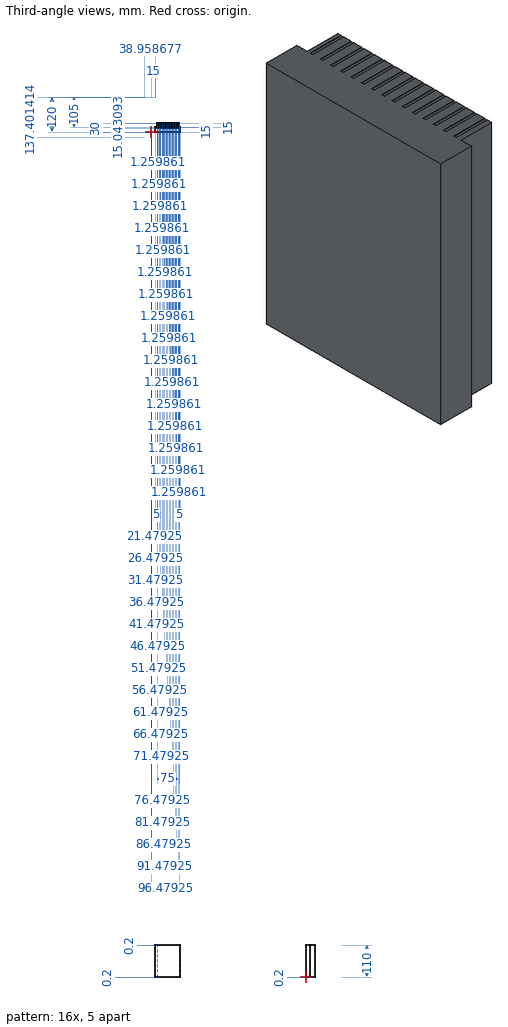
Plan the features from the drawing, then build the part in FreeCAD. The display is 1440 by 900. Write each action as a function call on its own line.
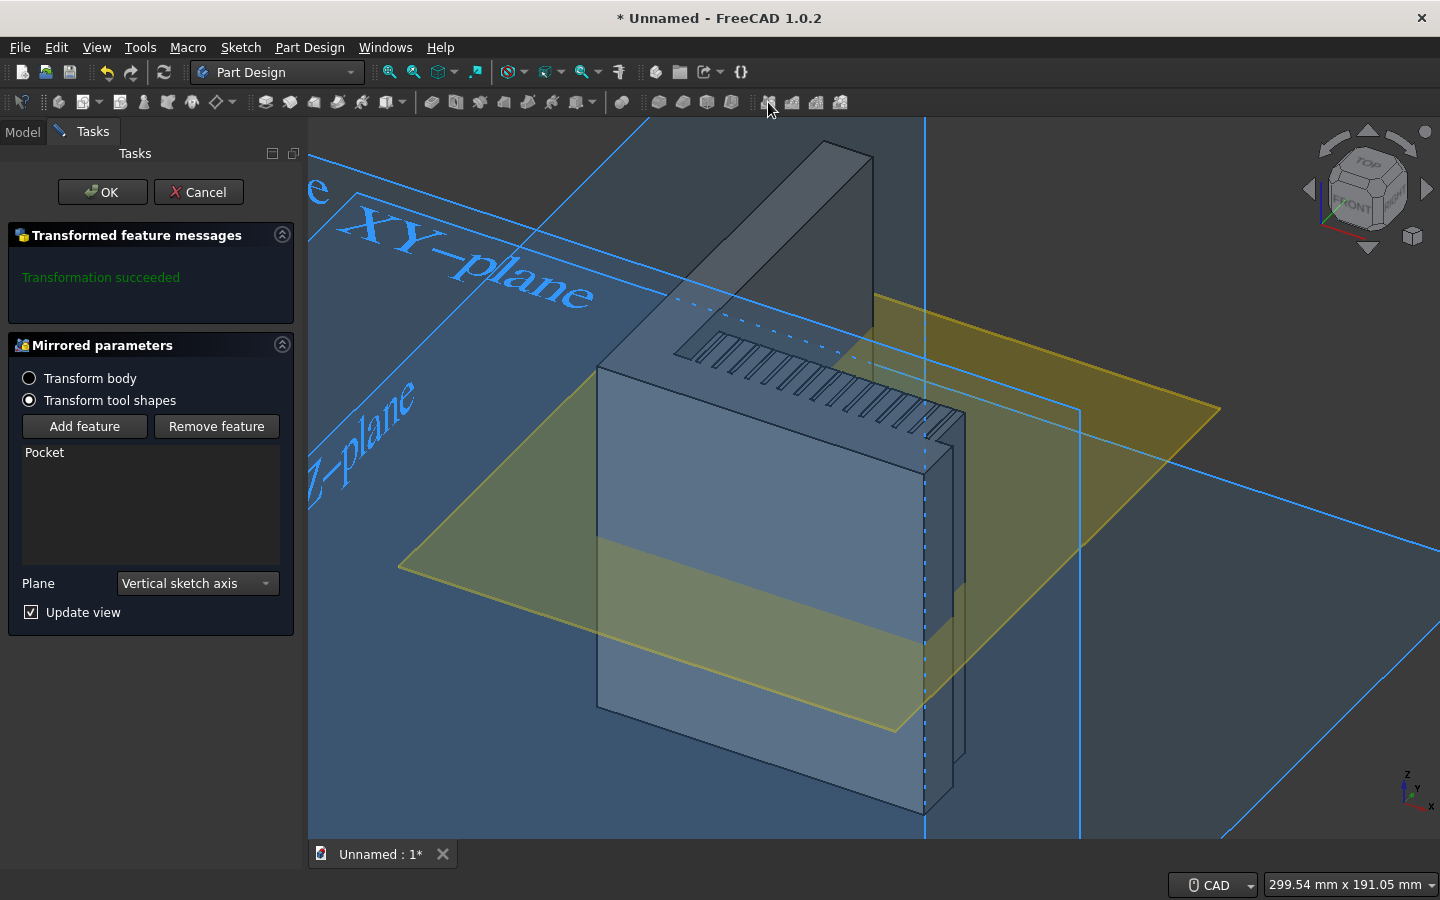
click(198, 584)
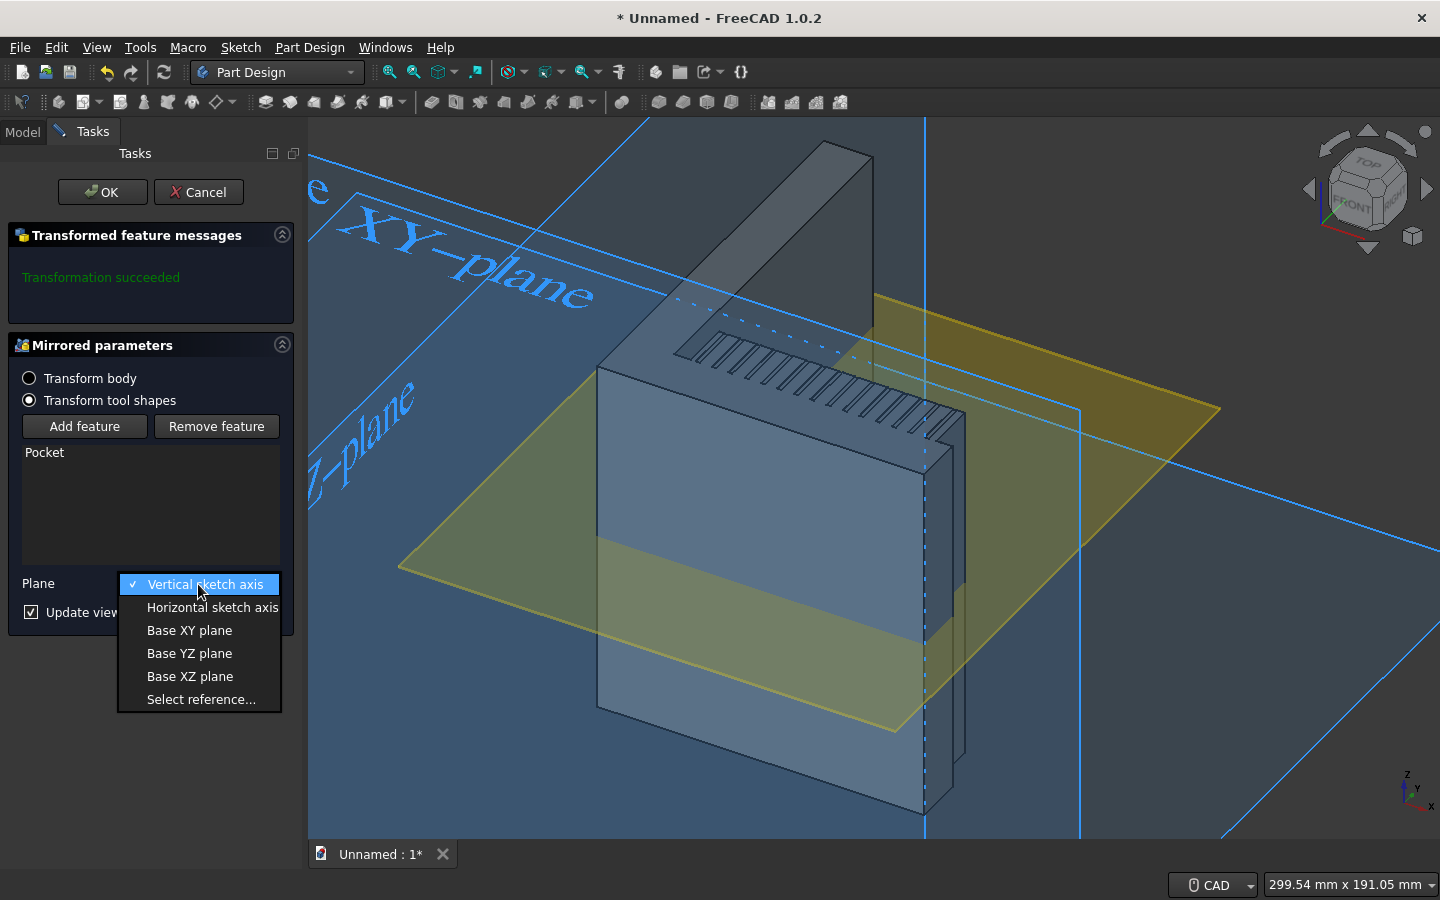
click(198, 700)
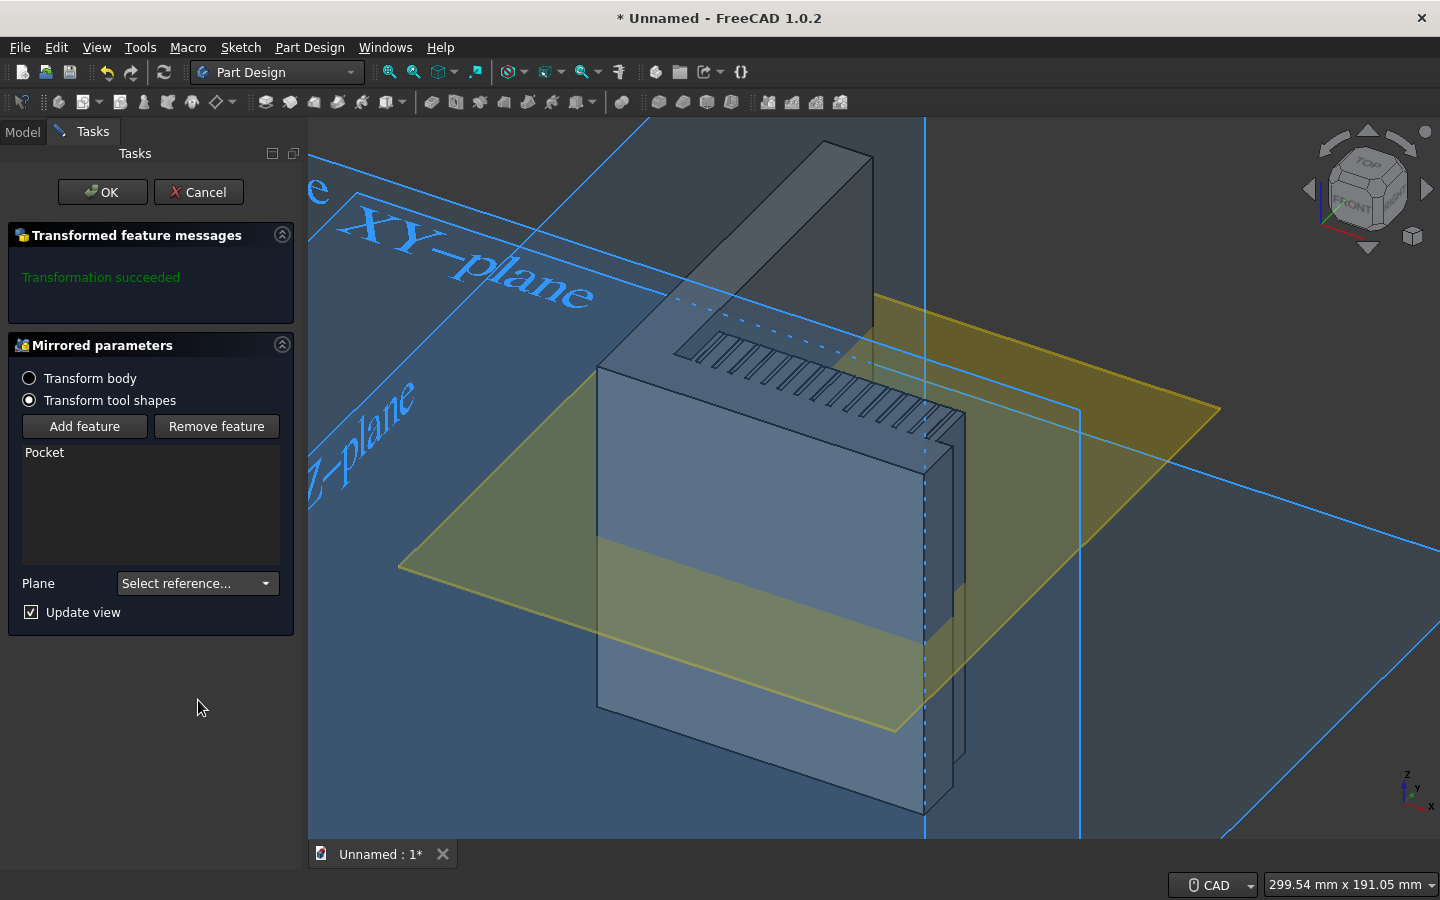
click(23, 131)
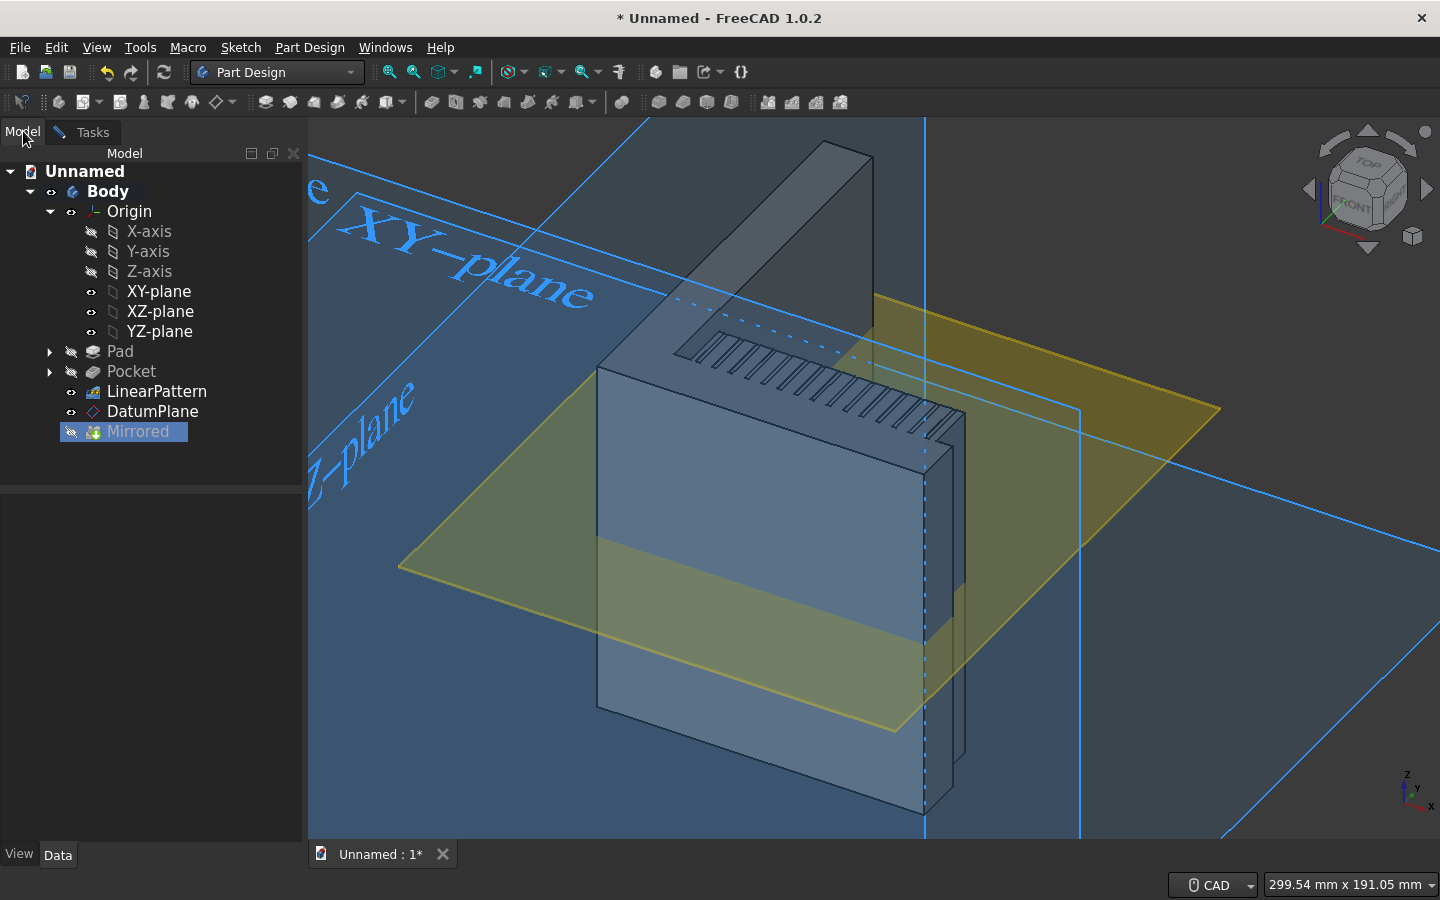
click(116, 412)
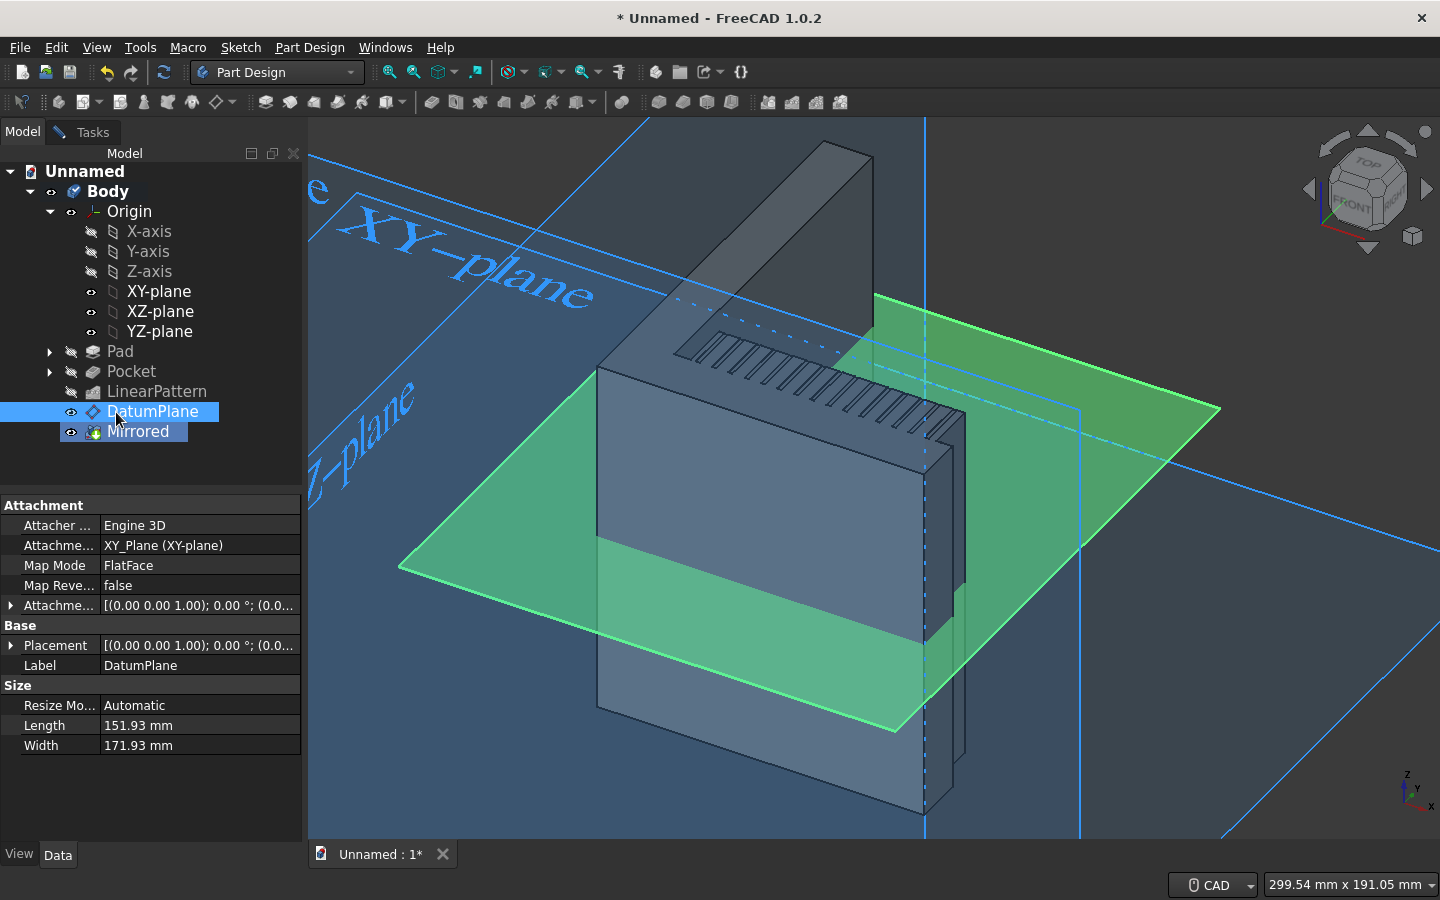
click(84, 131)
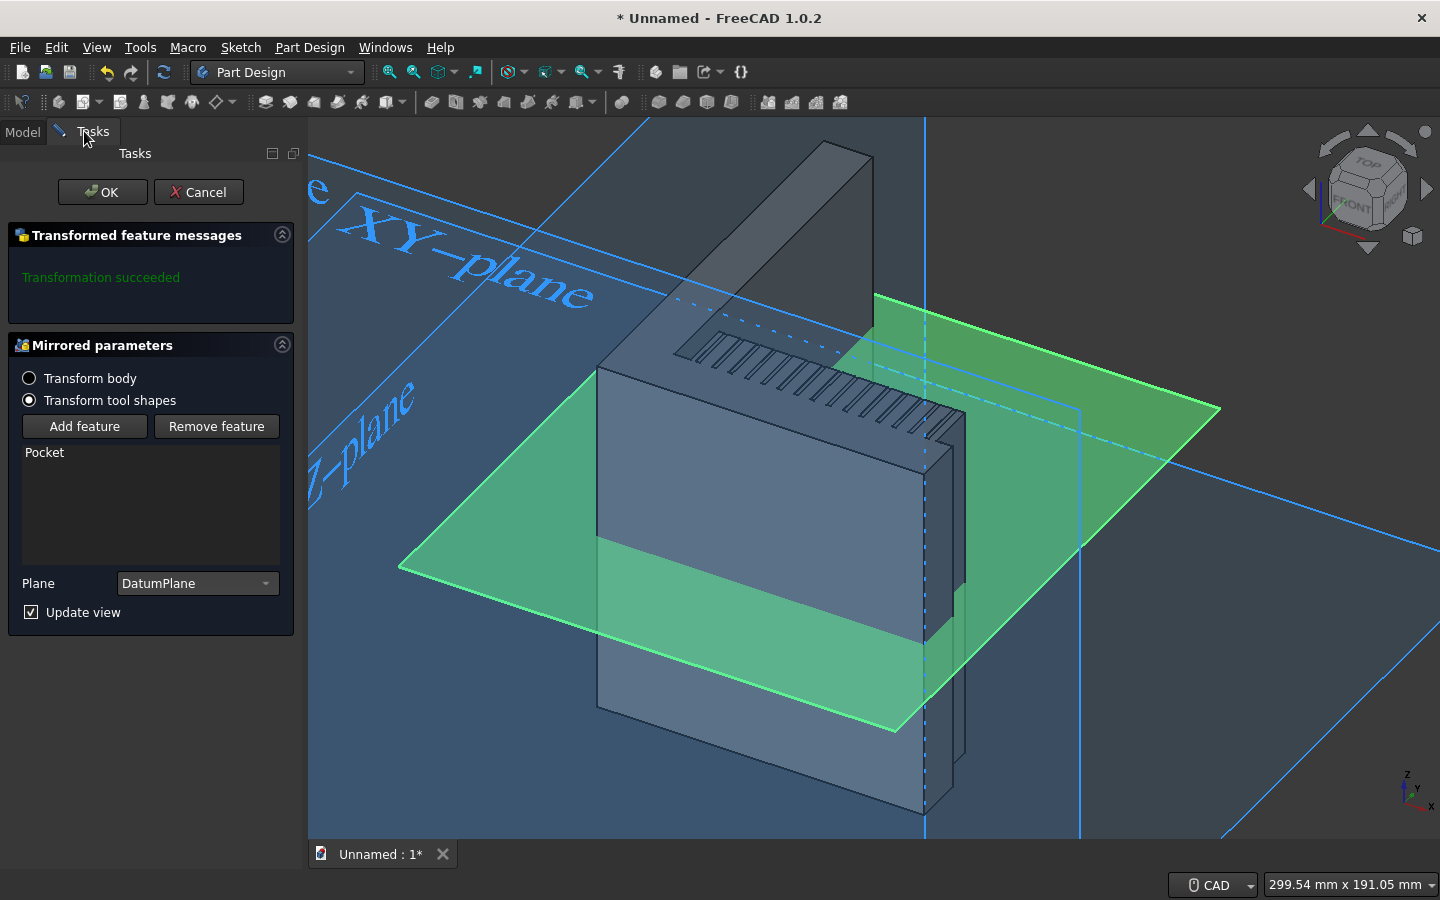
click(103, 192)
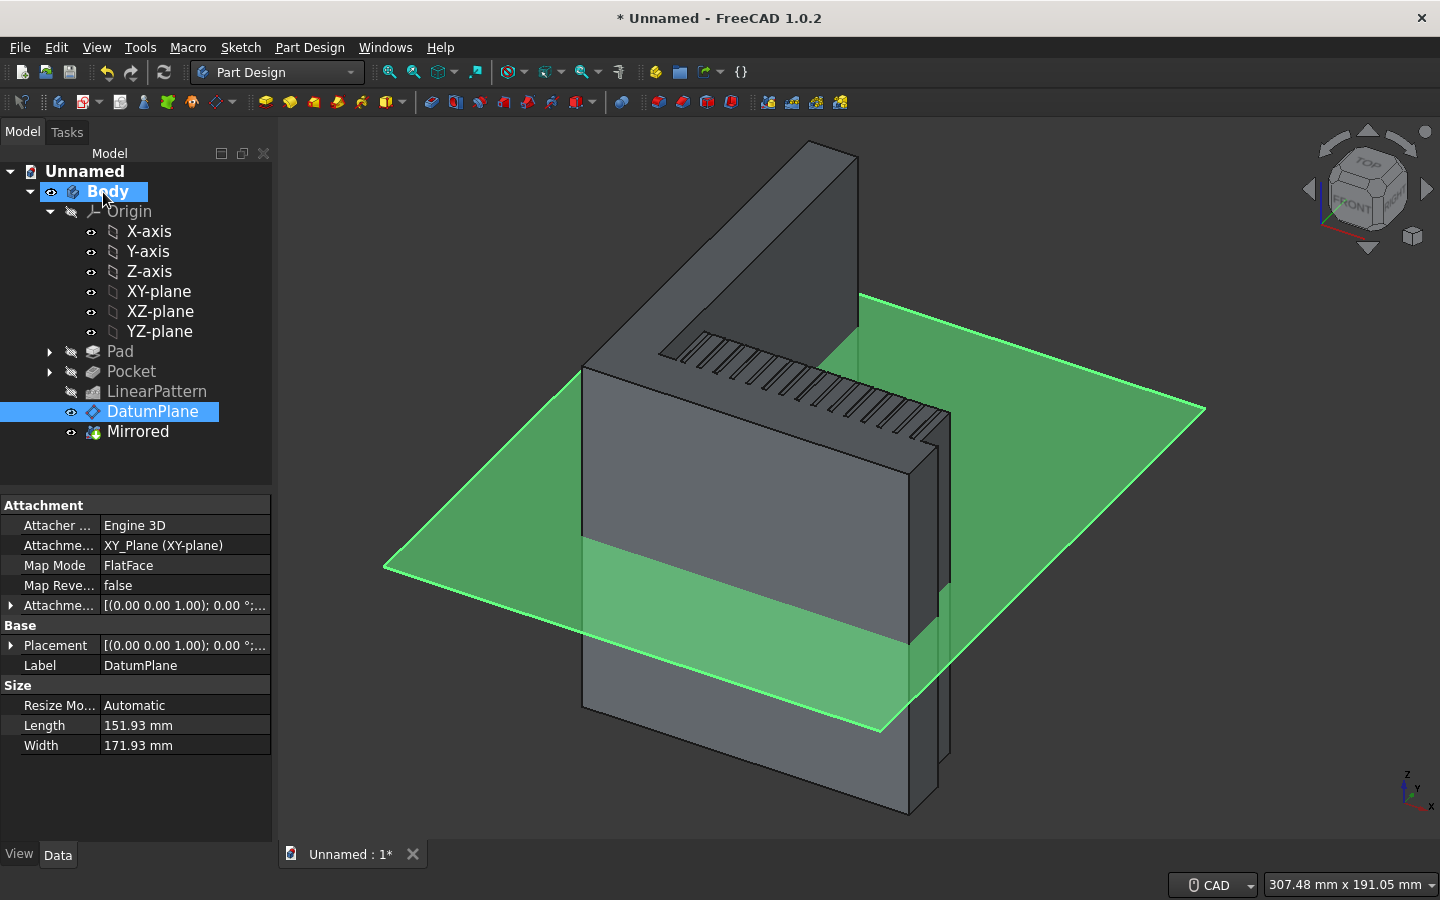
click(116, 412)
key(space)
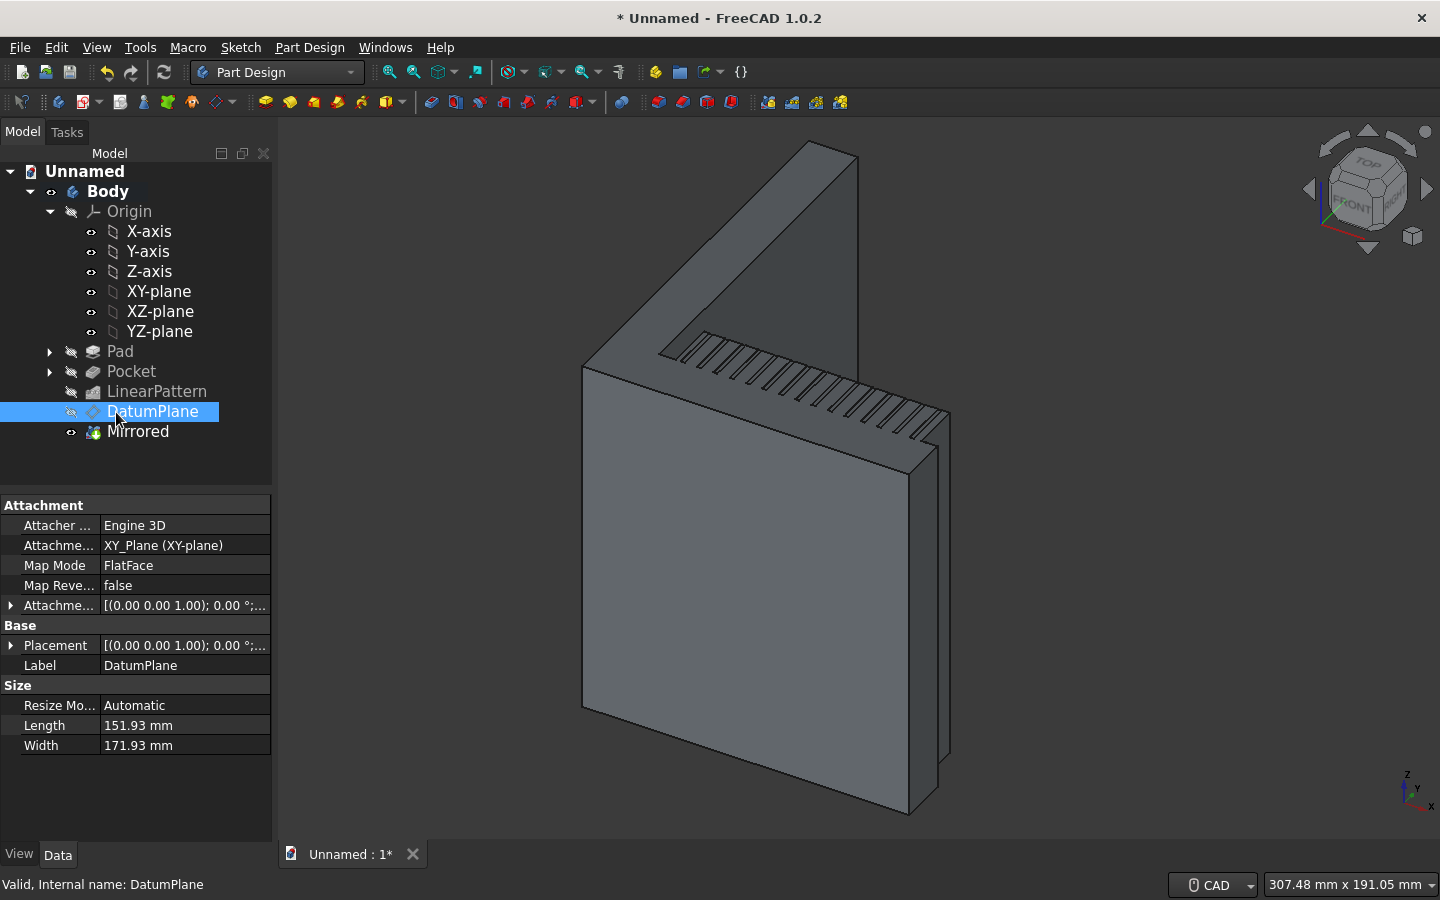
click(318, 799)